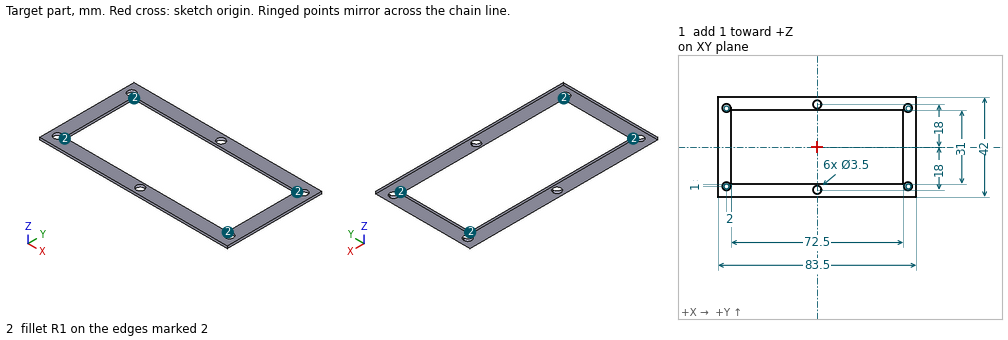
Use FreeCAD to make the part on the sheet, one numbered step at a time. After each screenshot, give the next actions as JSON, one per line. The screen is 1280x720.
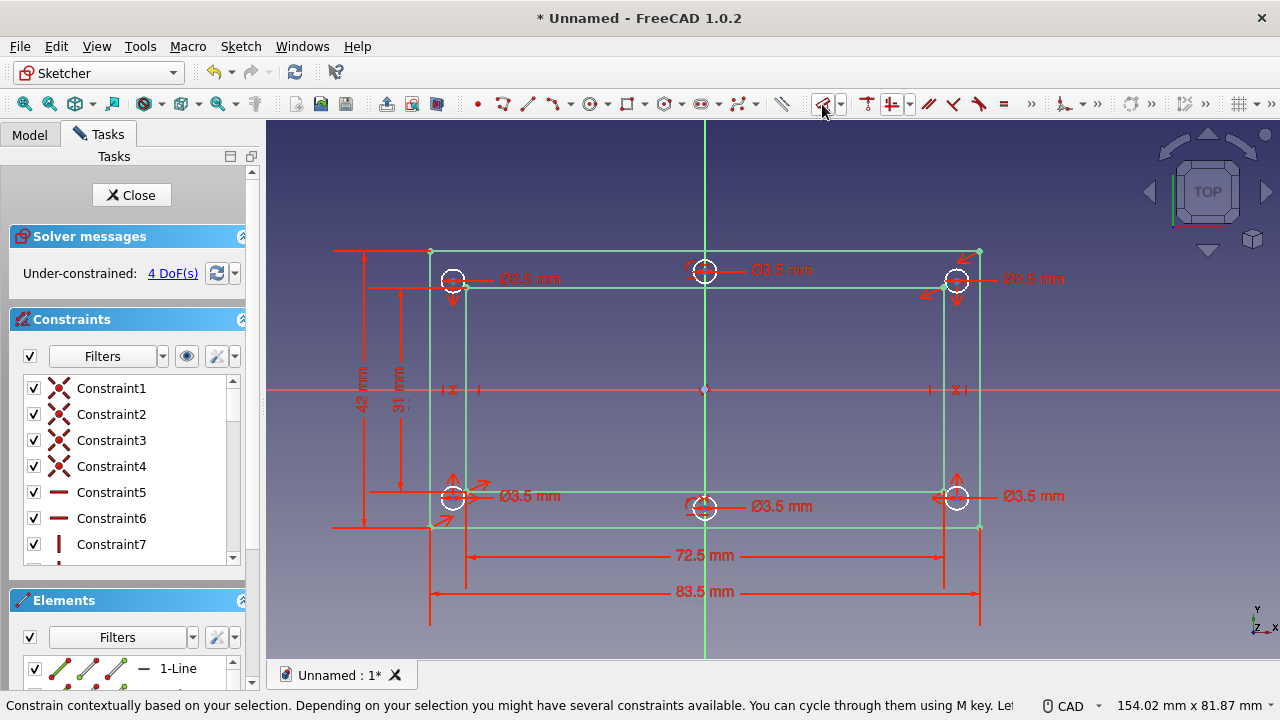
{"action": "left_click", "coordinate": [705, 508]}
{"action": "left_click", "coordinate": [739, 449]}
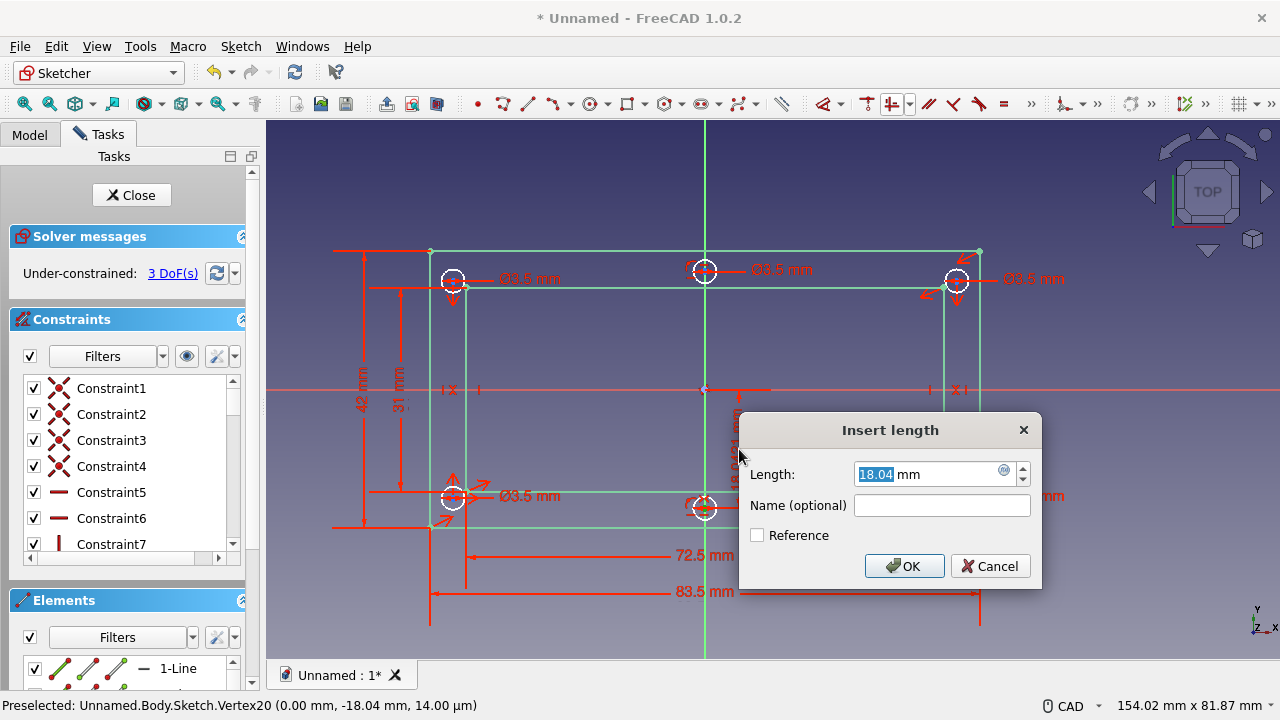
{"action": "type", "text": "18"}
{"action": "key", "text": "Return"}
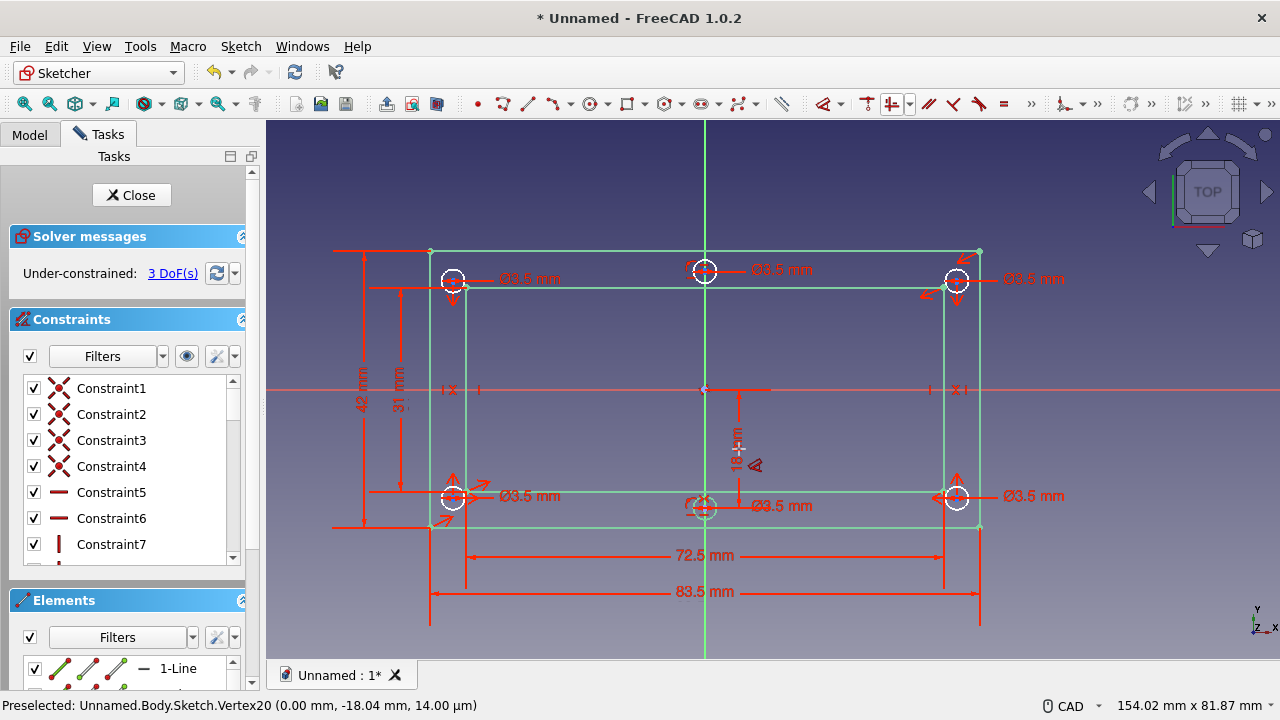
{"action": "left_click", "coordinate": [705, 272]}
{"action": "left_click", "coordinate": [739, 331]}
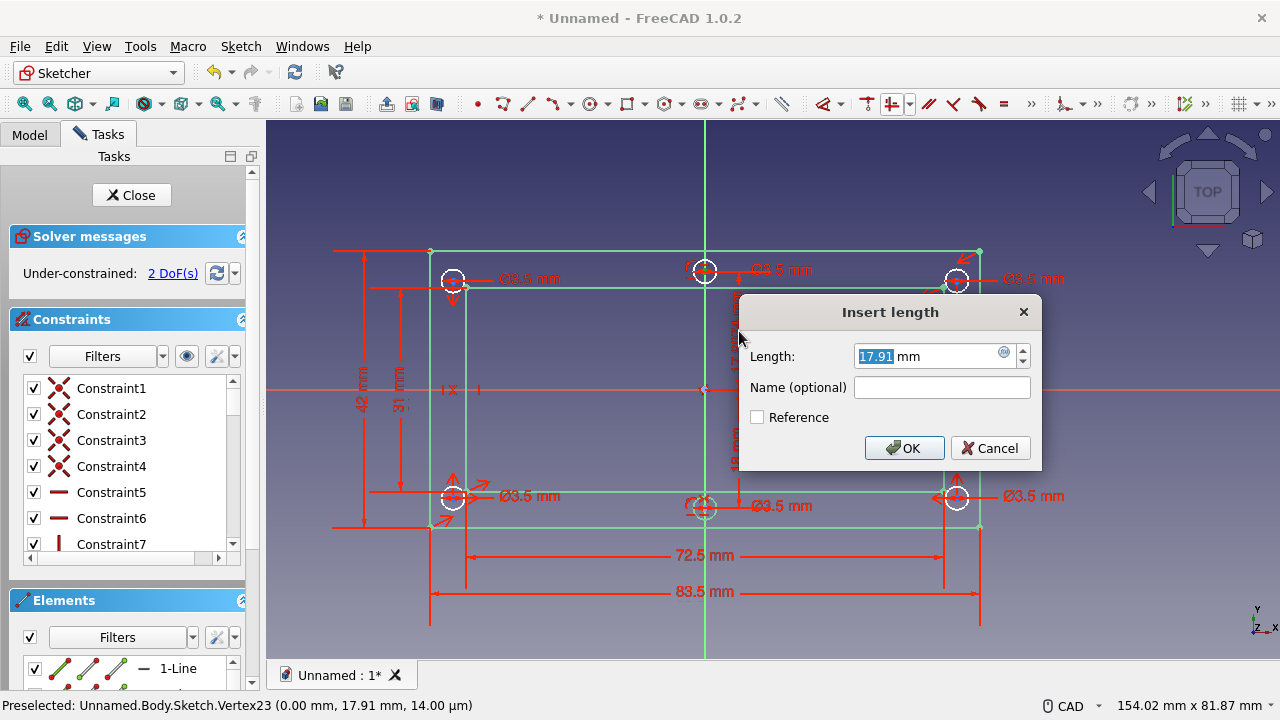
{"action": "type", "text": "18"}
{"action": "key", "text": "Return"}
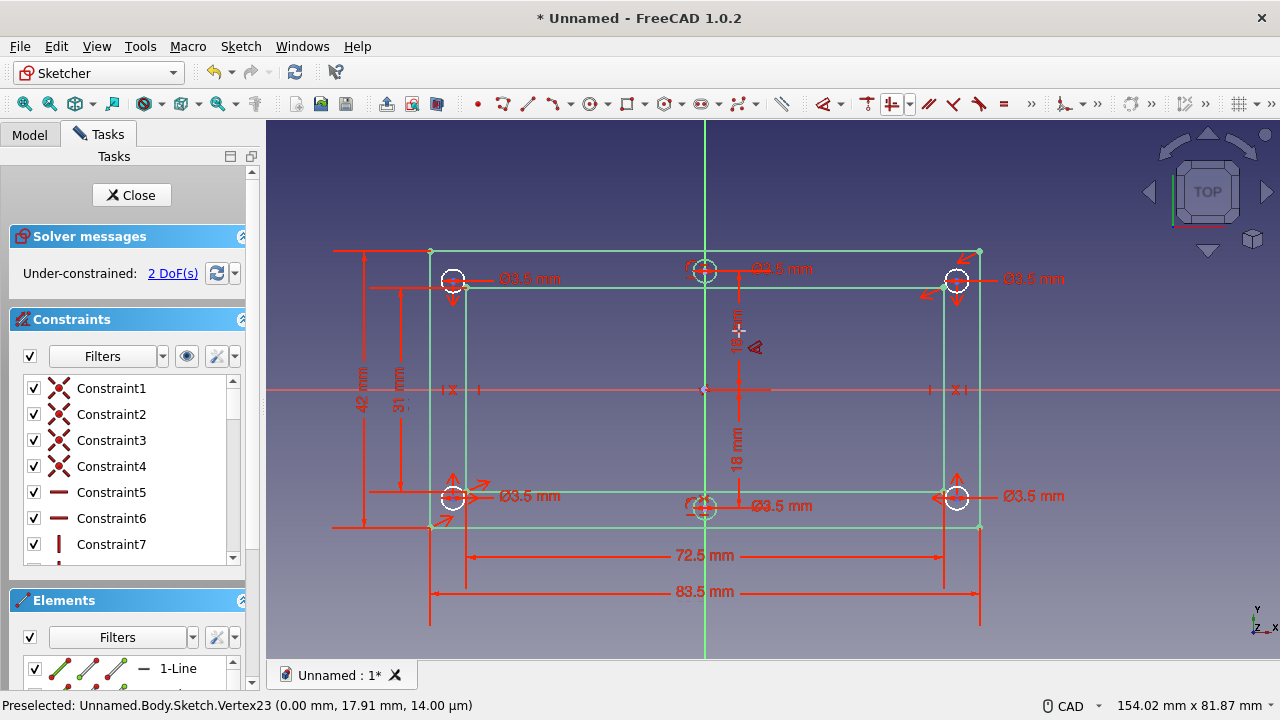
{"action": "scroll", "coordinate": [466, 492], "scroll_direction": "up", "scroll_amount": 6}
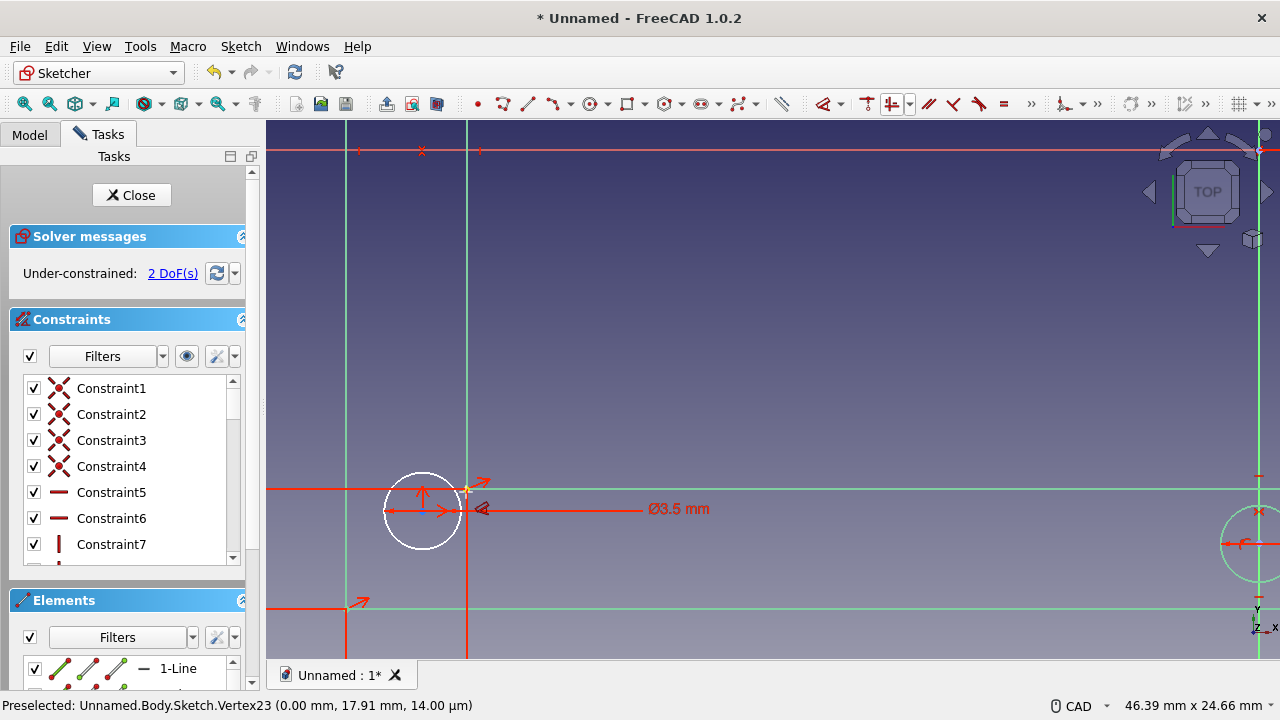
{"action": "left_click", "coordinate": [467, 489]}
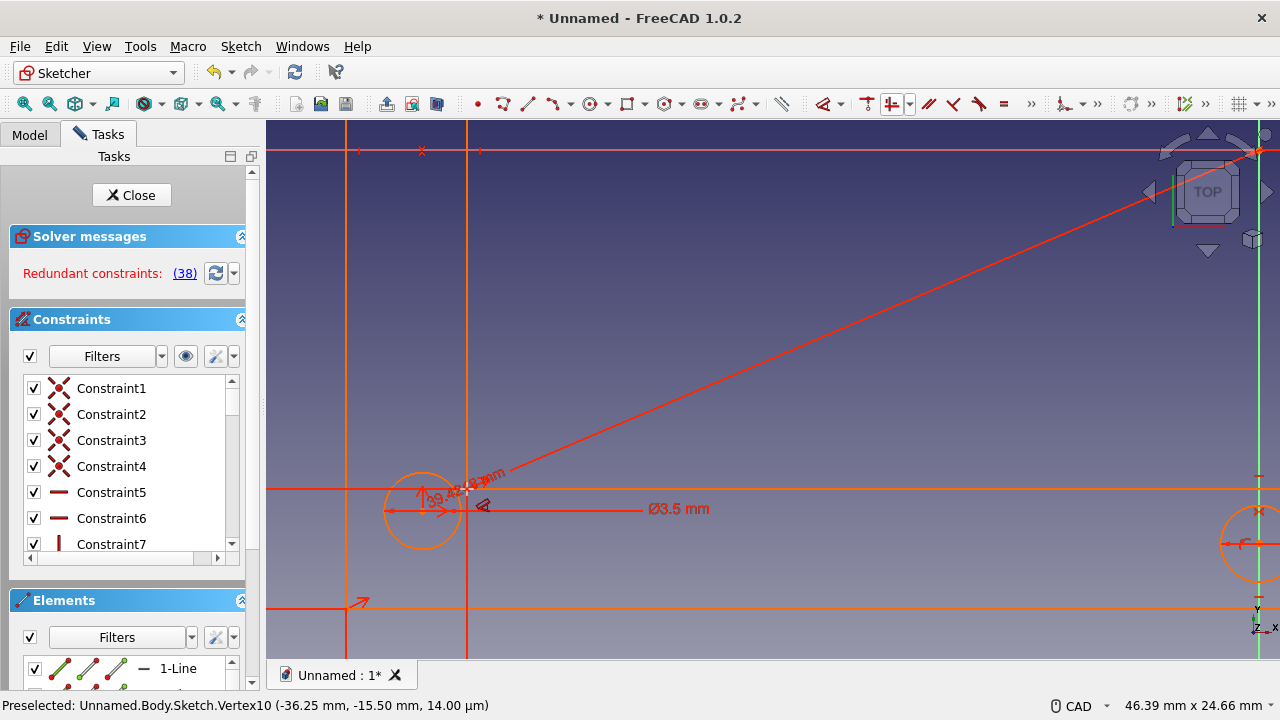
{"action": "left_click", "coordinate": [423, 511]}
{"action": "left_click", "coordinate": [445, 455]}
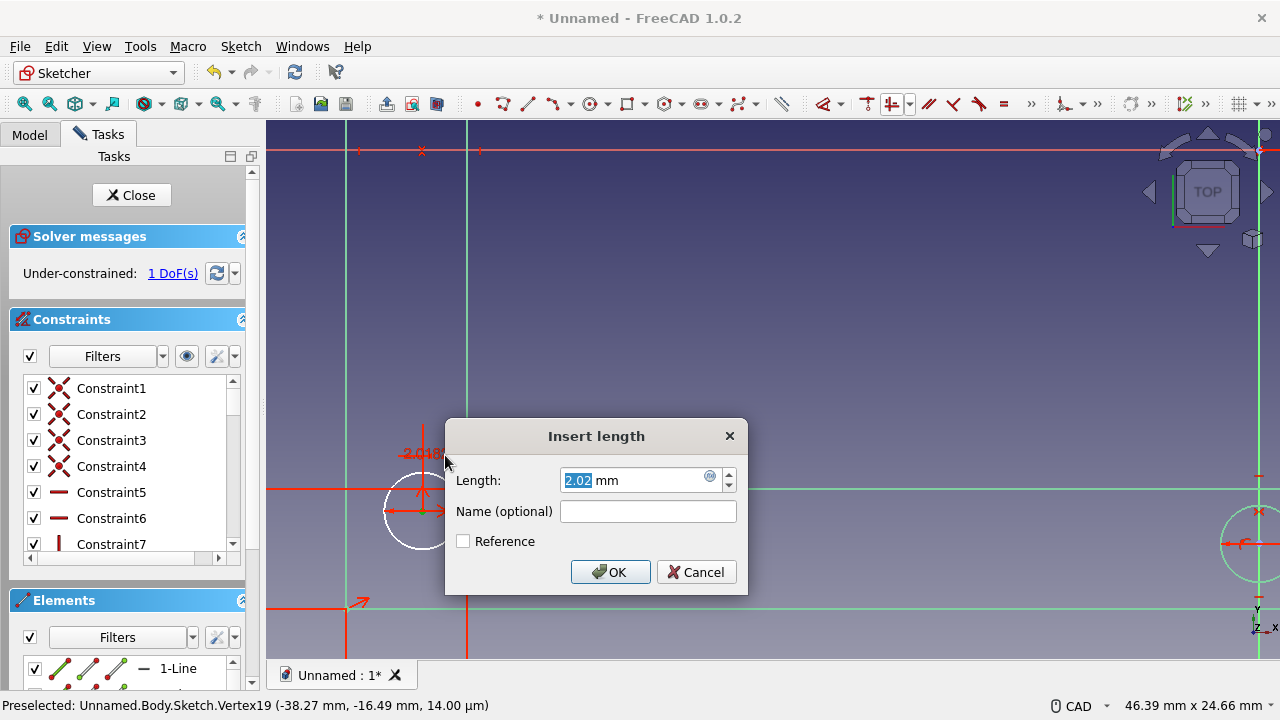
{"action": "type", "text": "2"}
{"action": "key", "text": "Return"}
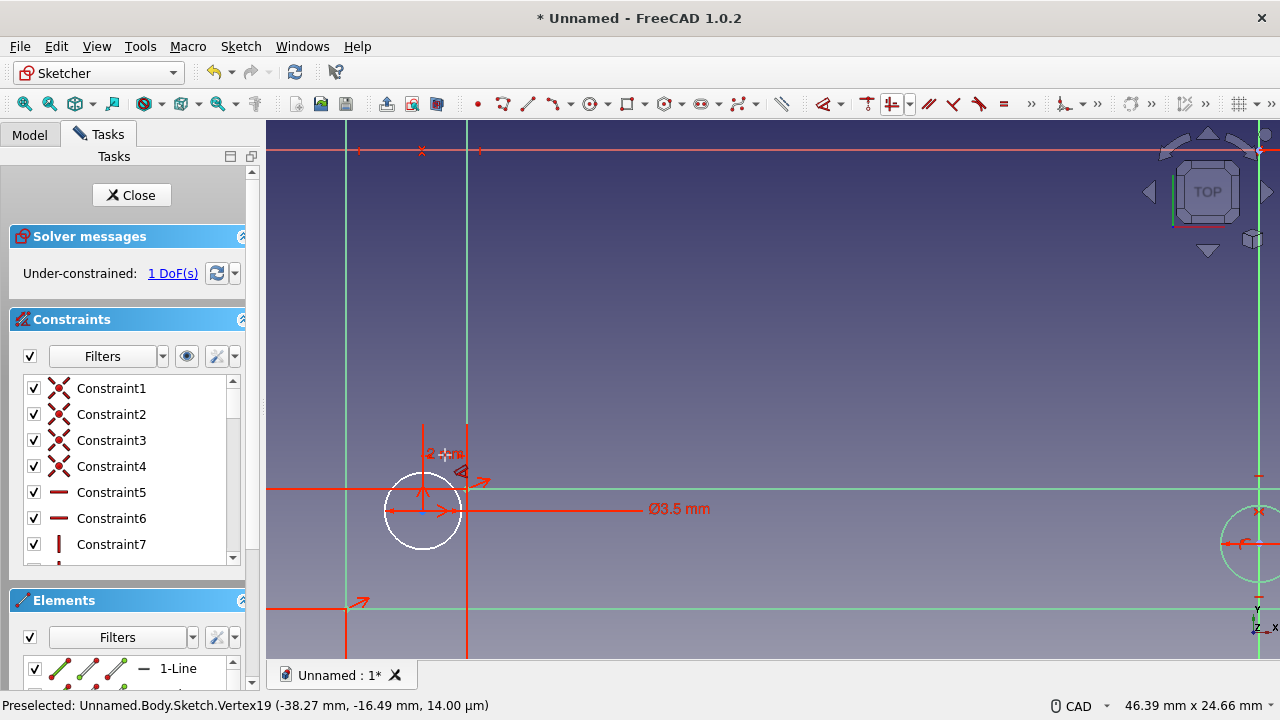
{"action": "scroll", "coordinate": [467, 489], "scroll_direction": "up", "scroll_amount": 3}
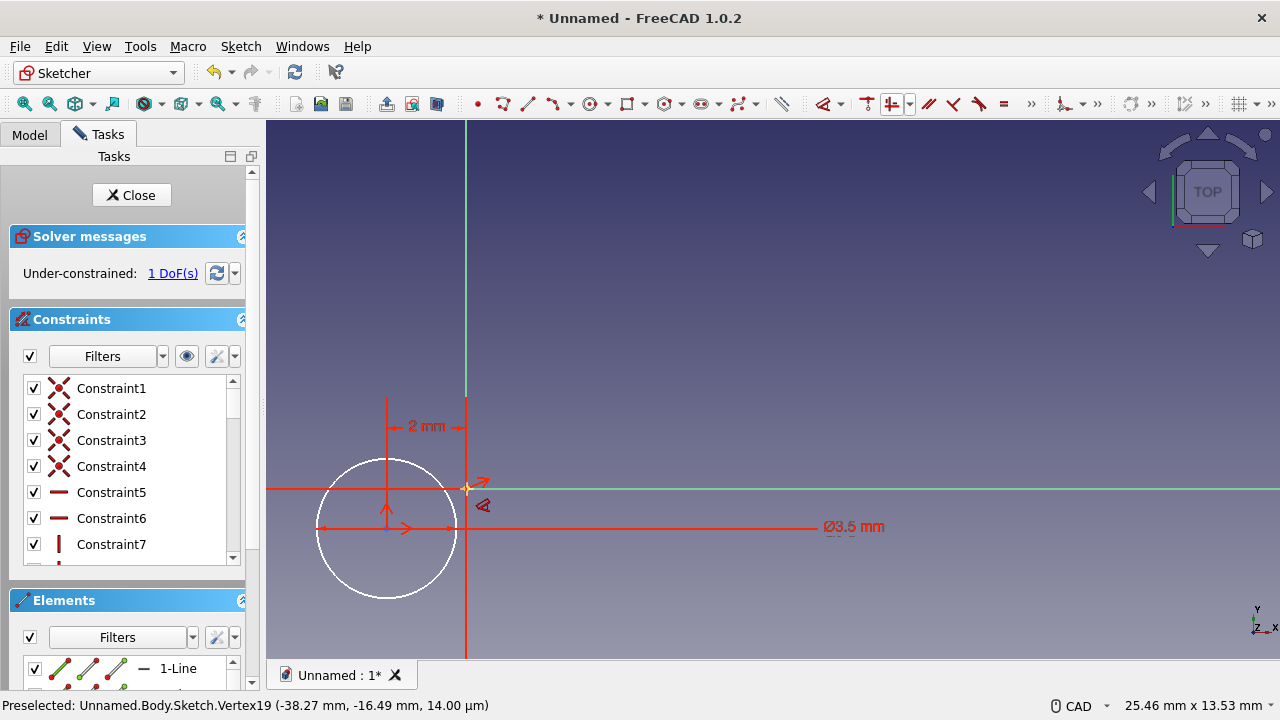
{"action": "left_click", "coordinate": [466, 489]}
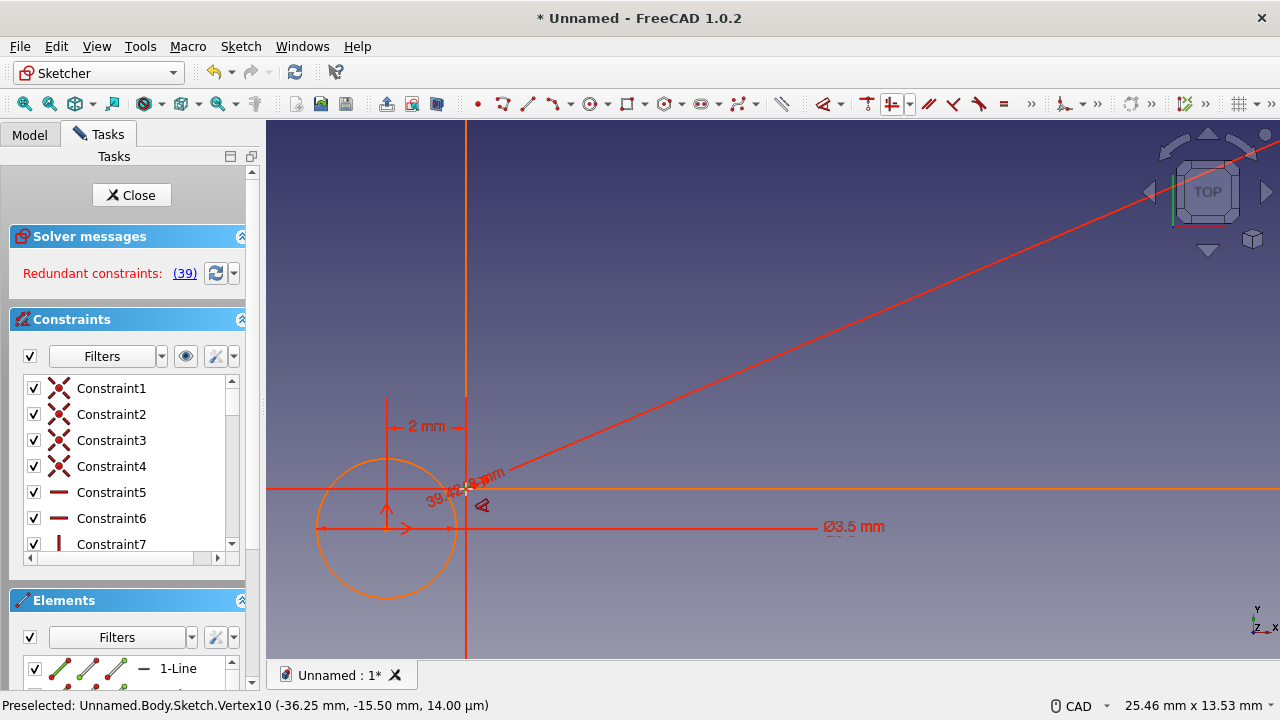
{"action": "left_click", "coordinate": [387, 529]}
{"action": "left_click", "coordinate": [353, 509]}